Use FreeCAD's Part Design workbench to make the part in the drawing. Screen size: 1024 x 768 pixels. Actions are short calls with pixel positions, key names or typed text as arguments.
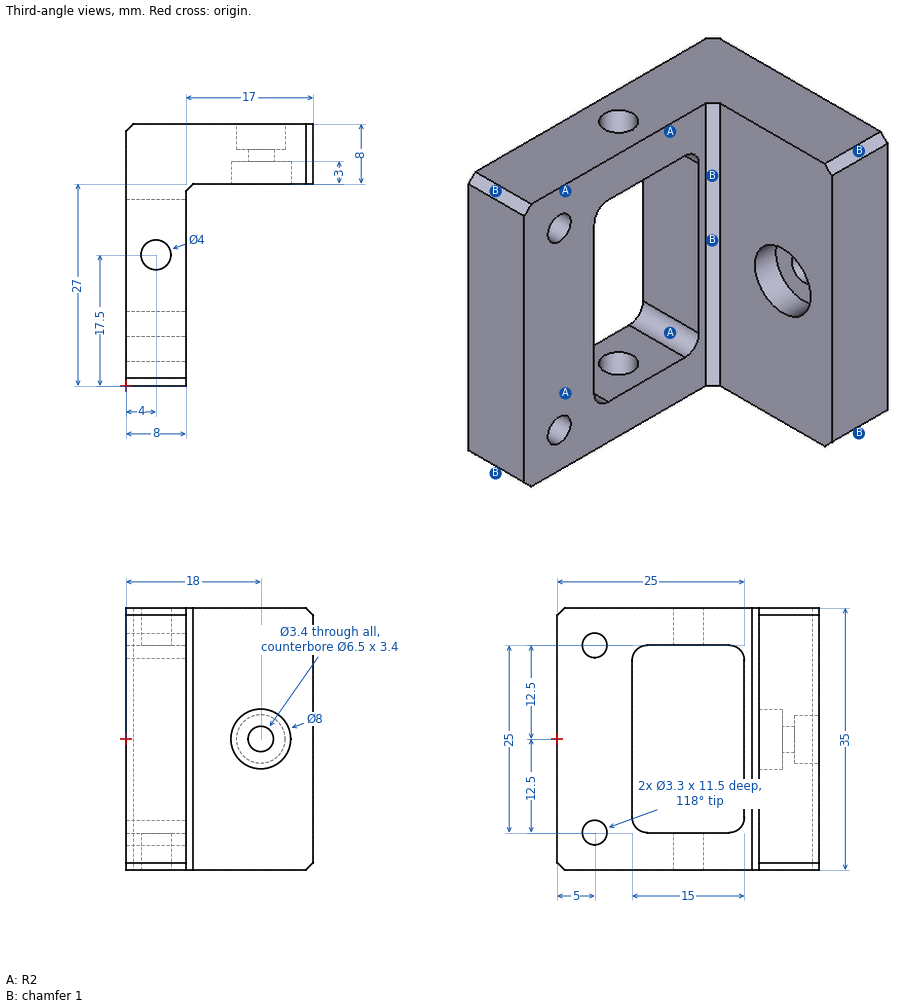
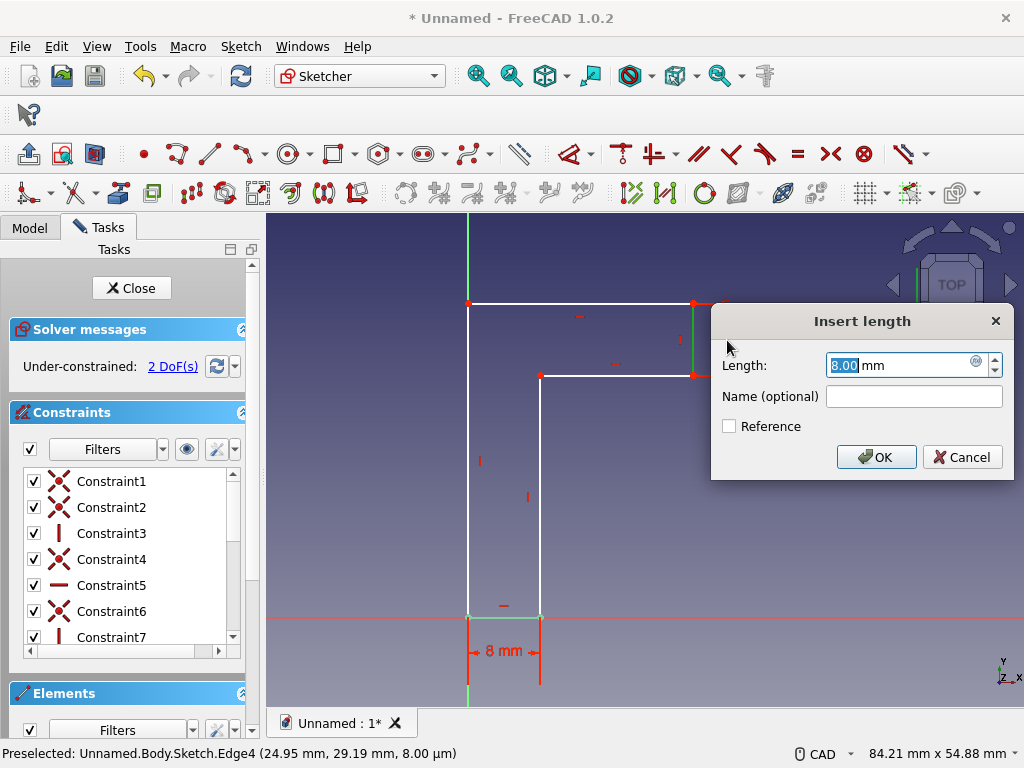
text(8)
key(Return)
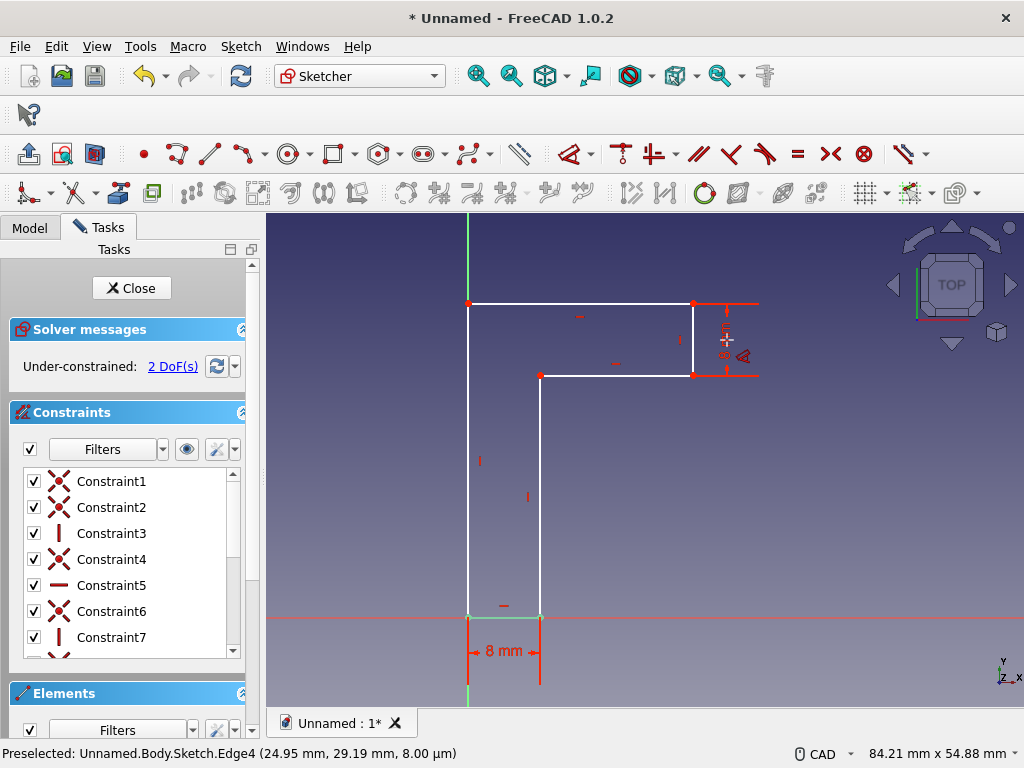
click(540, 545)
click(506, 497)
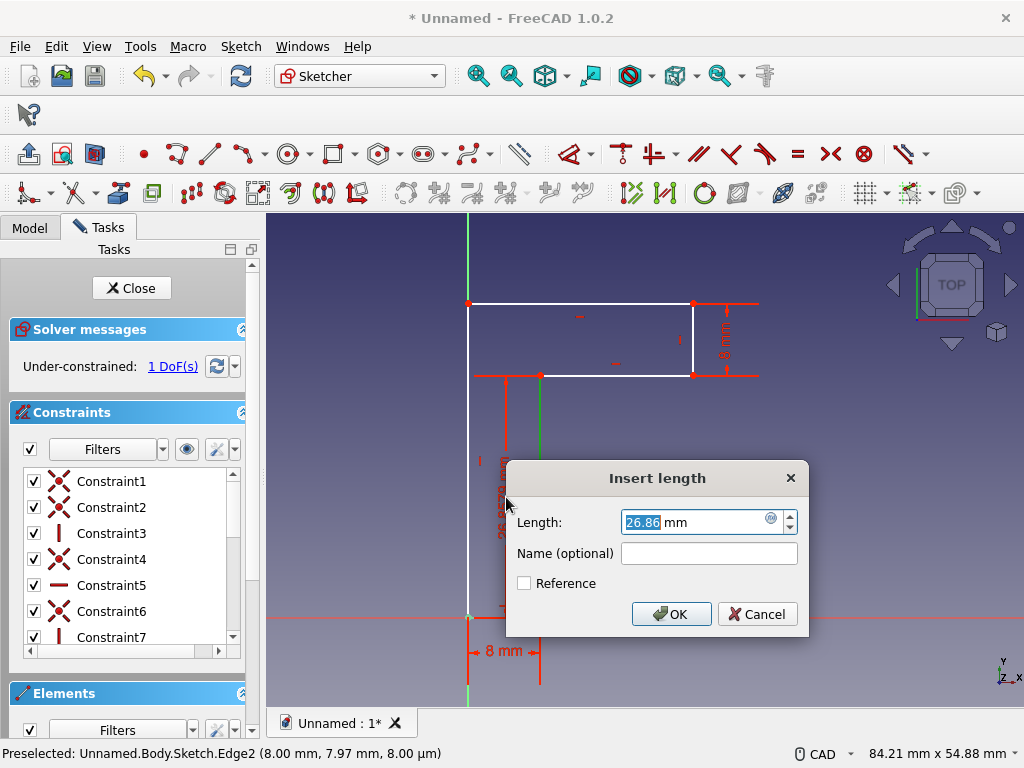
text(27)
key(Return)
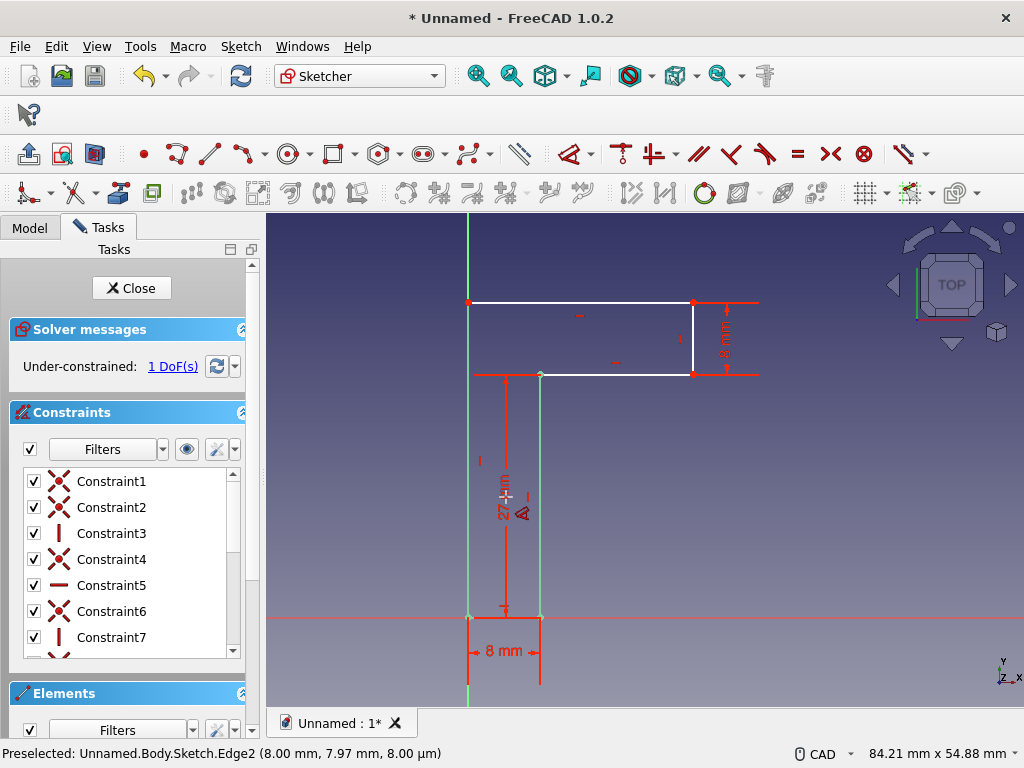
click(586, 375)
click(617, 341)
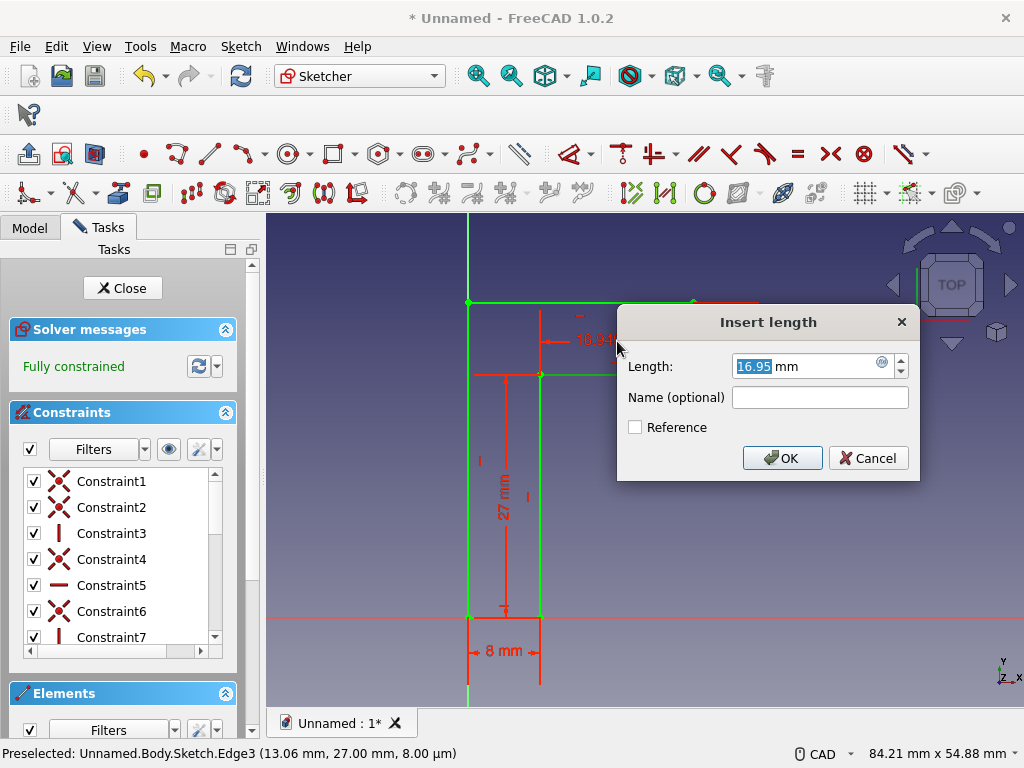
text(17)
key(Return)
key(Escape)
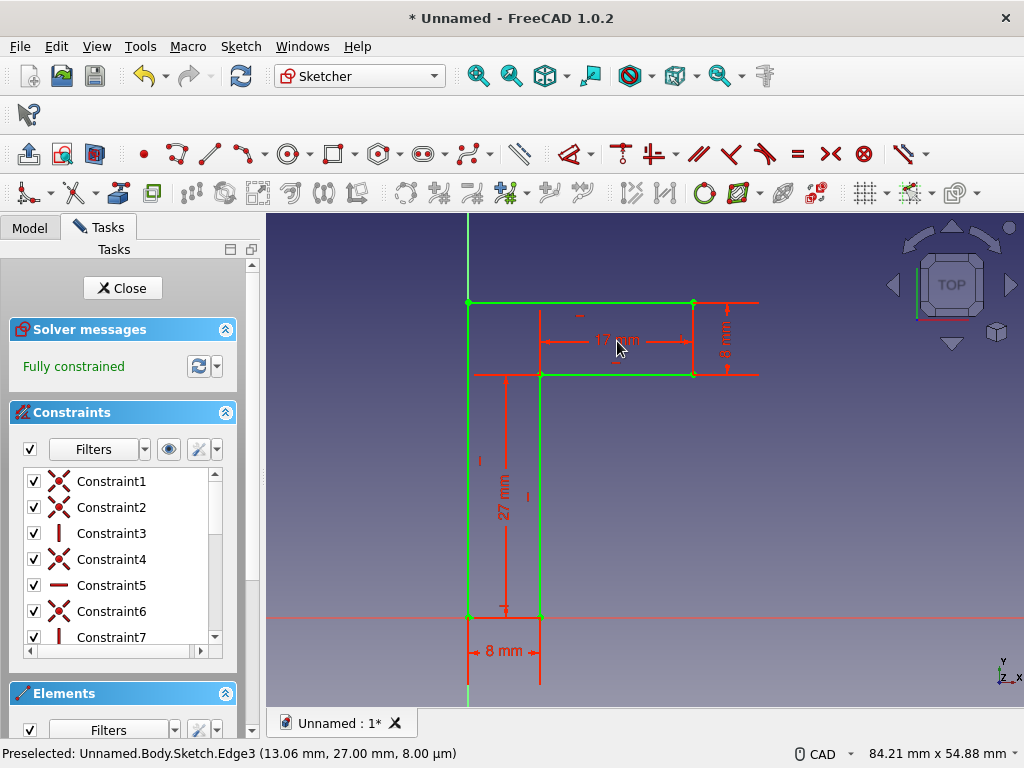
click(123, 288)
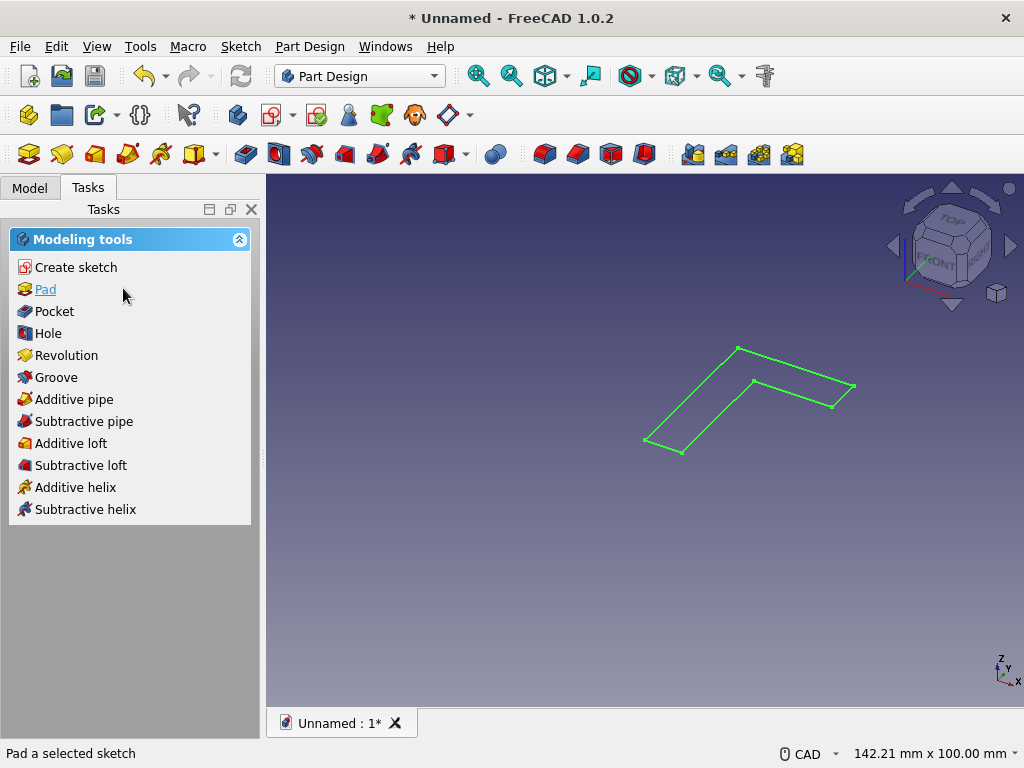
click(29, 154)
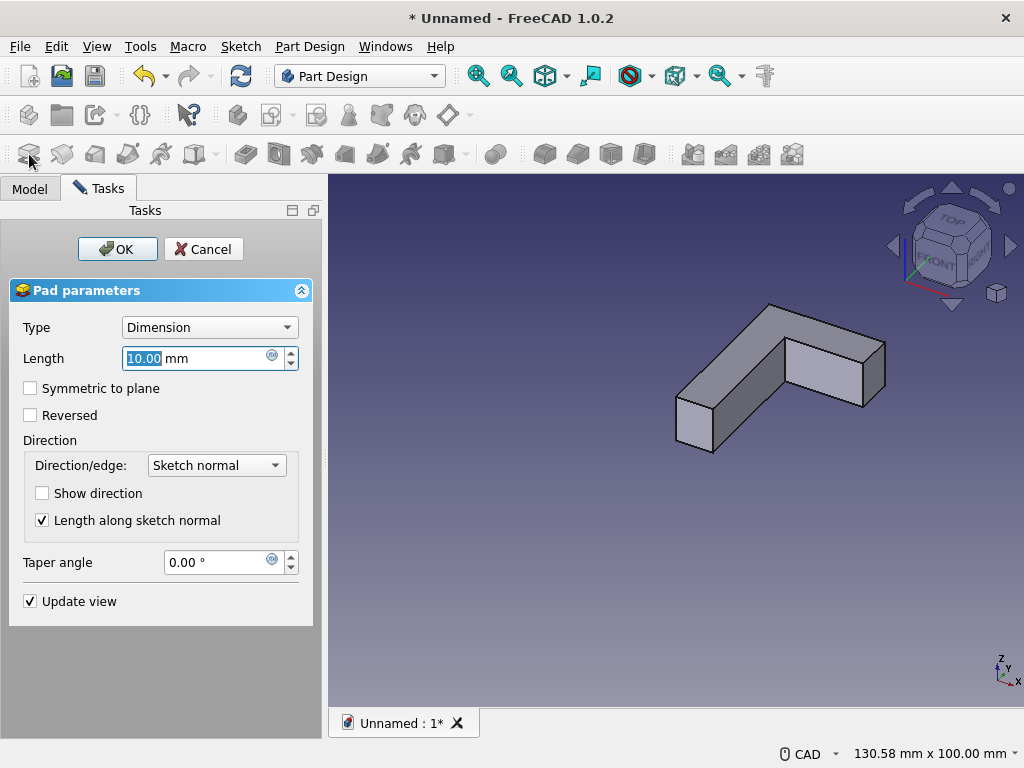
text(35)
key(Tab)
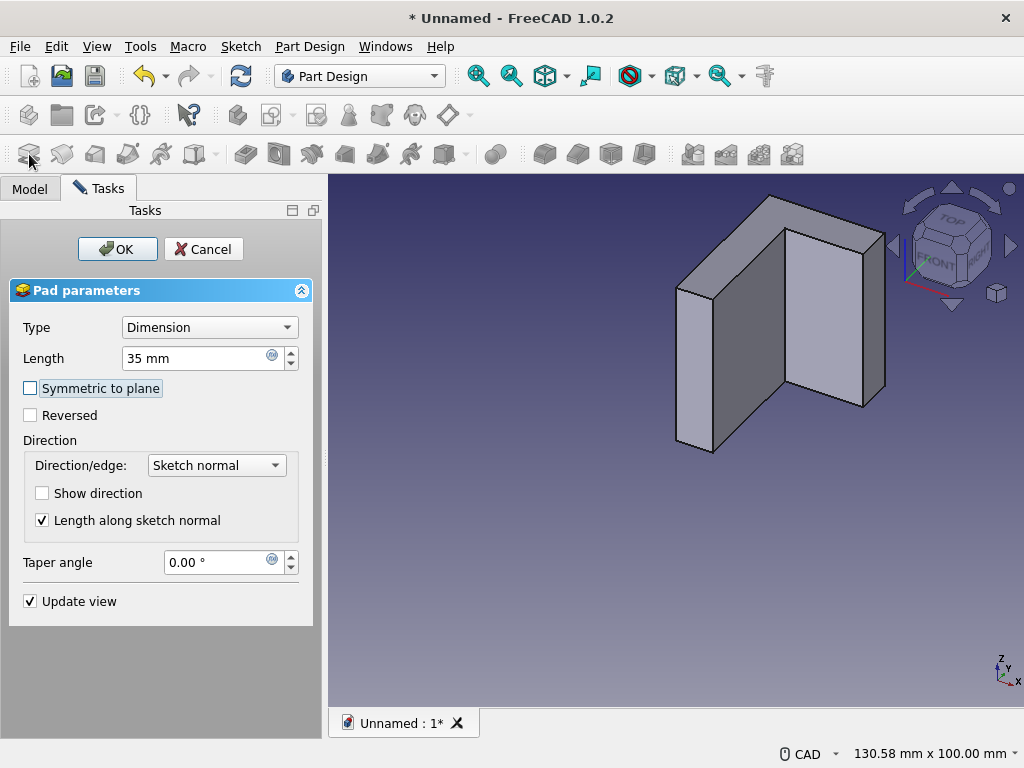
click(31, 388)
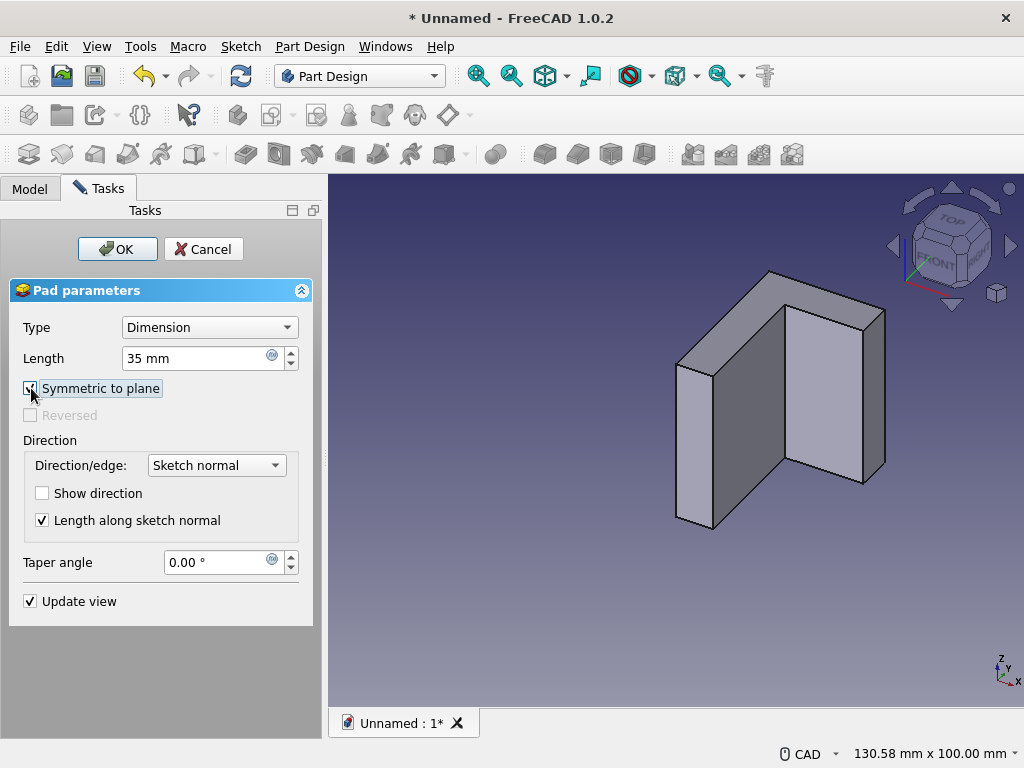
click(118, 249)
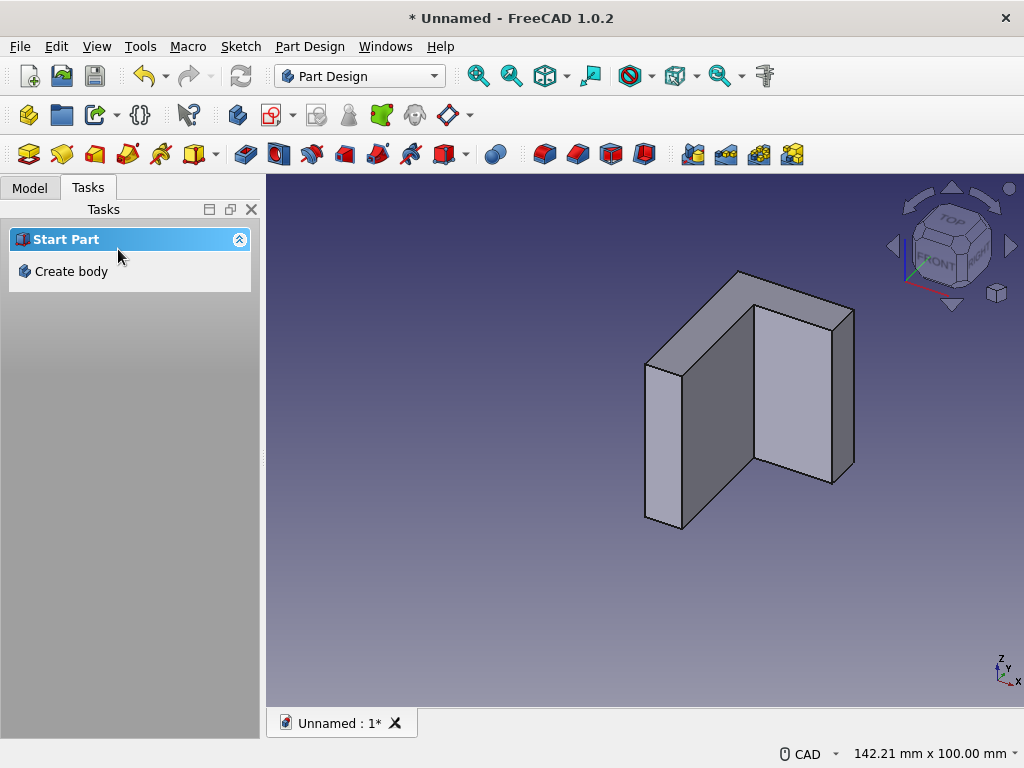
key(6)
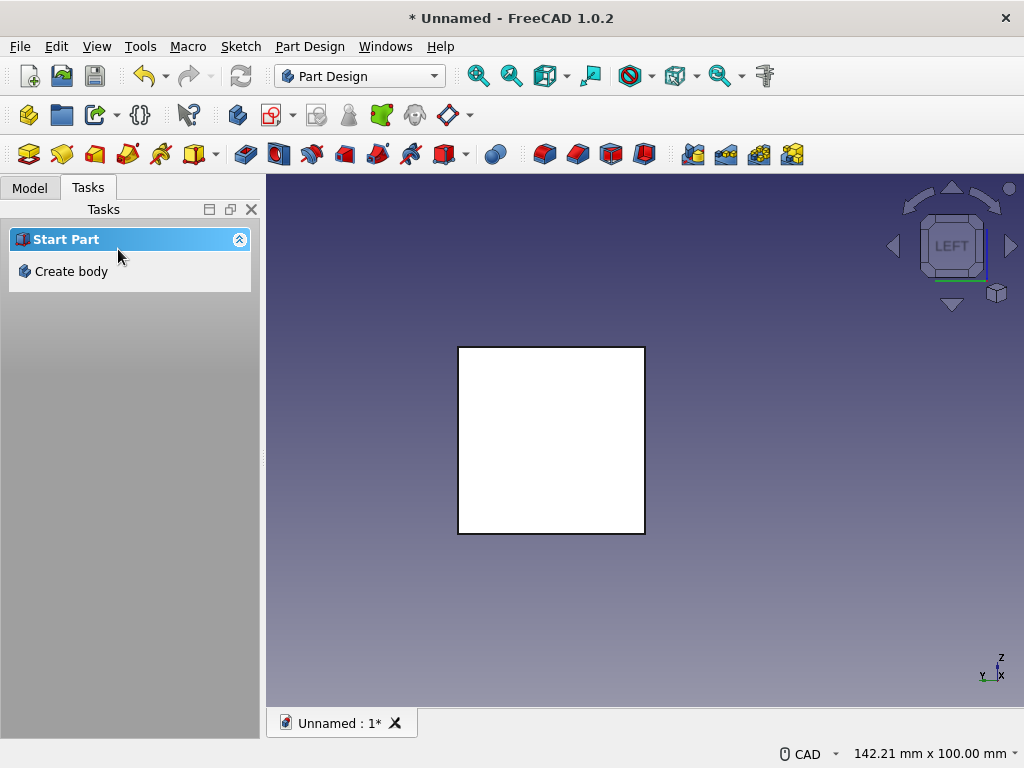
key(v)
key(f)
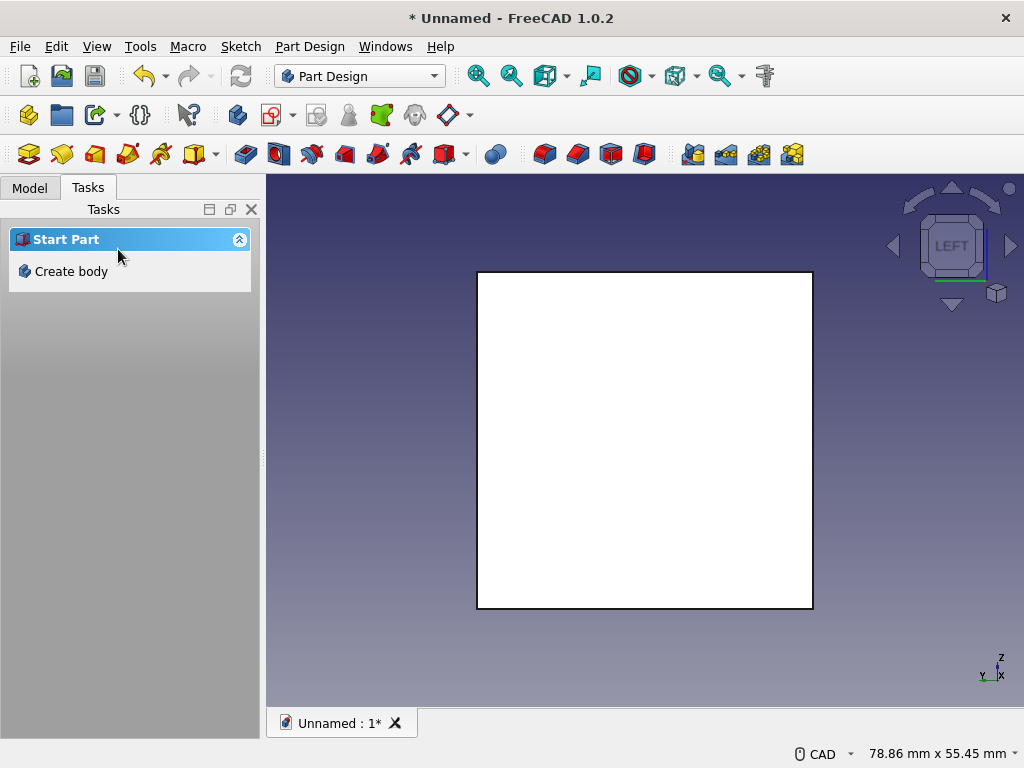
click(645, 439)